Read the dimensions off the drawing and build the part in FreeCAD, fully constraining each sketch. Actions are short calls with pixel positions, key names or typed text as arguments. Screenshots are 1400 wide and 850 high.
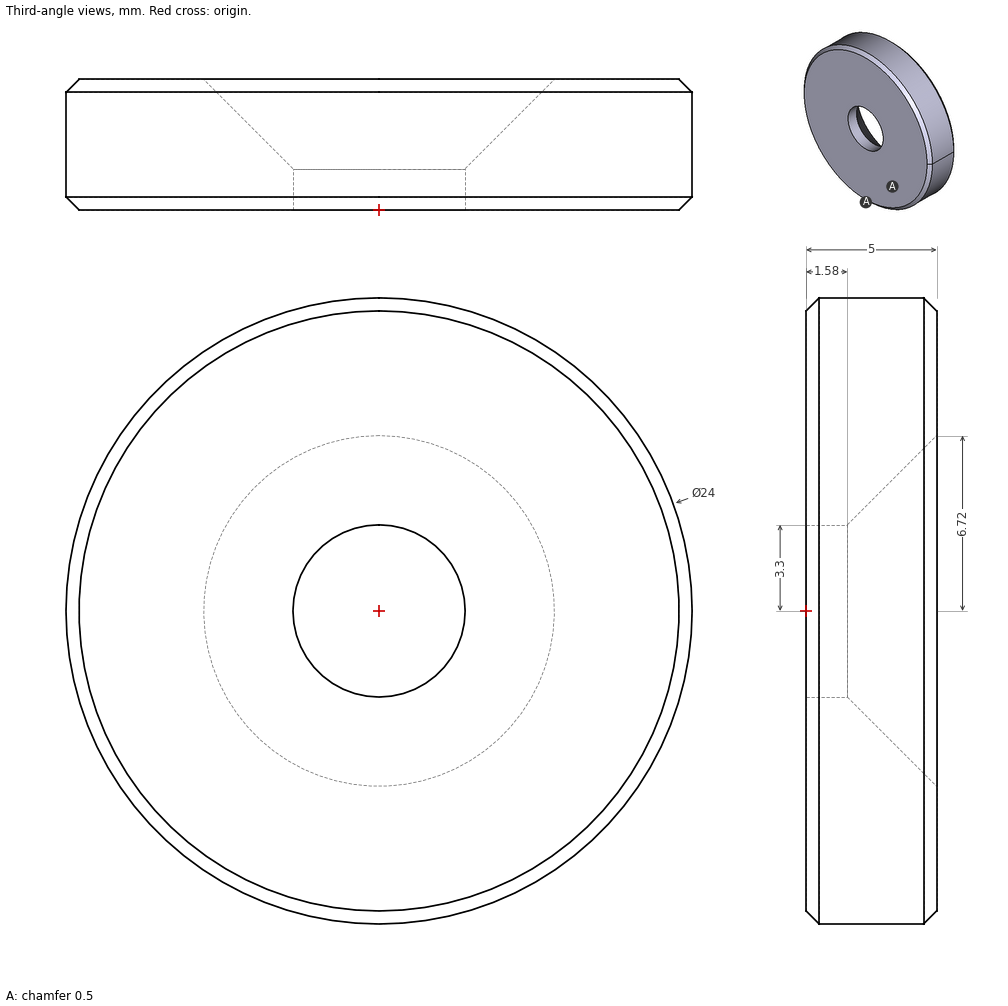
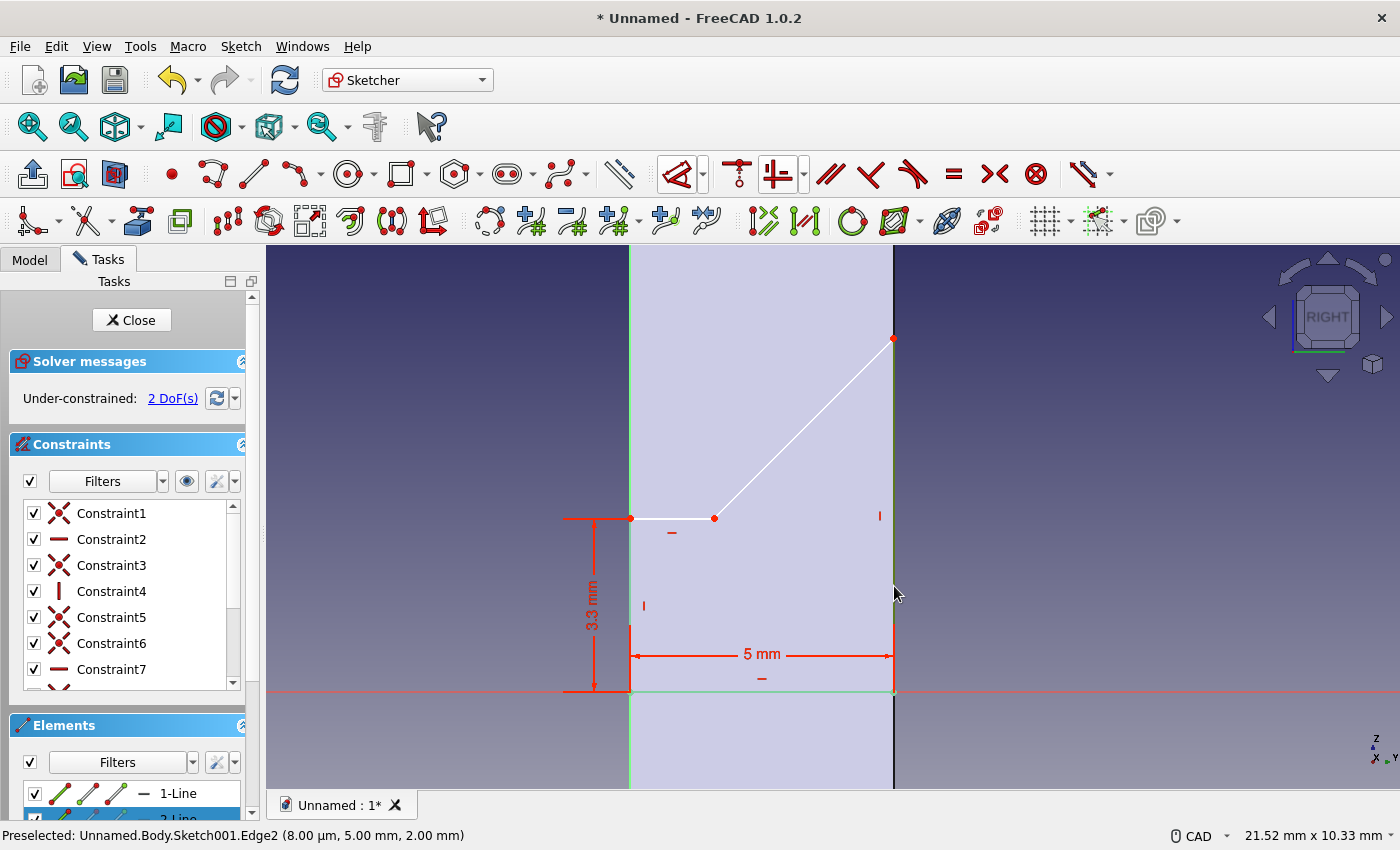
key(i)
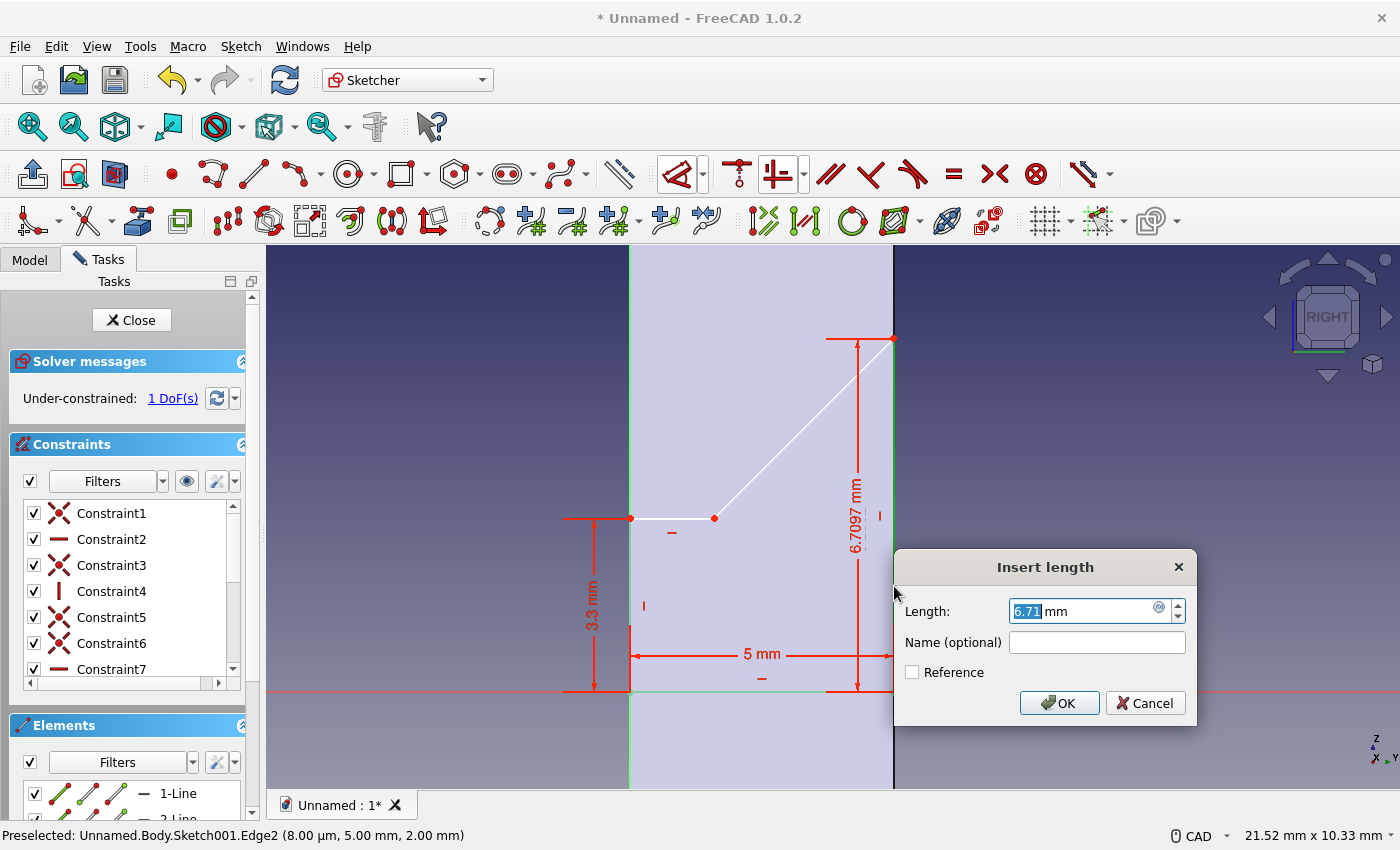
text(6.72)
key(Return)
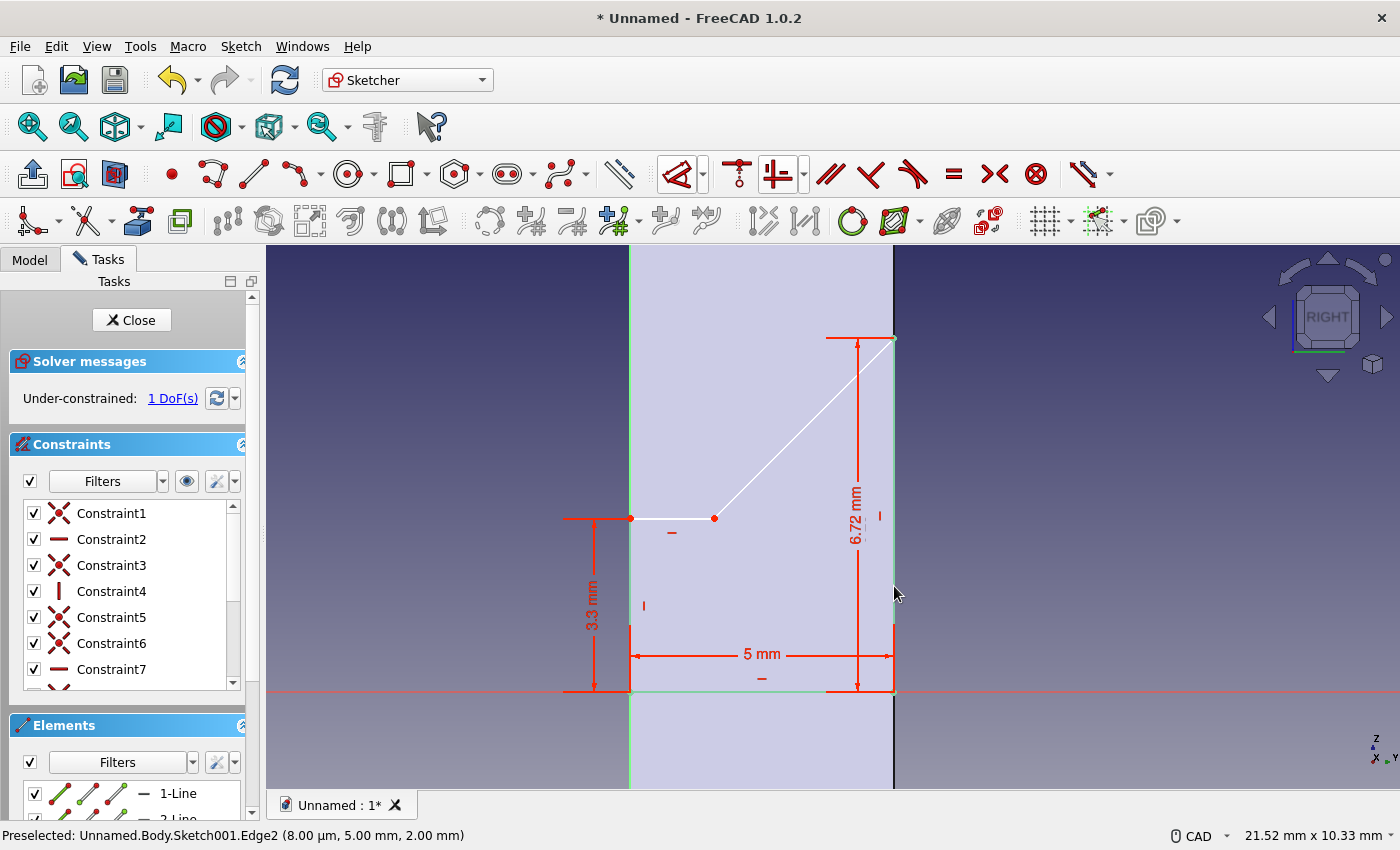
click(689, 519)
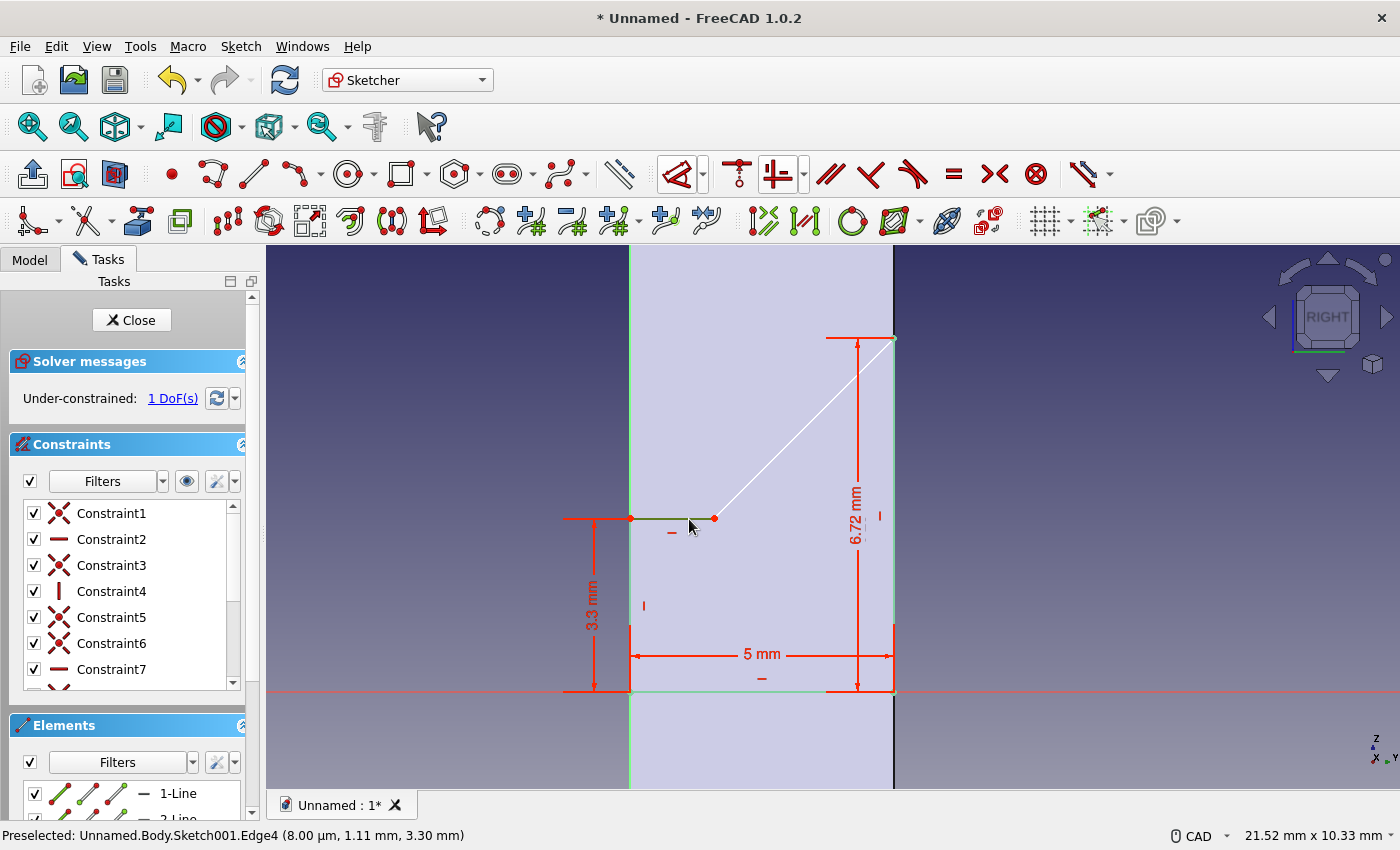
click(702, 174)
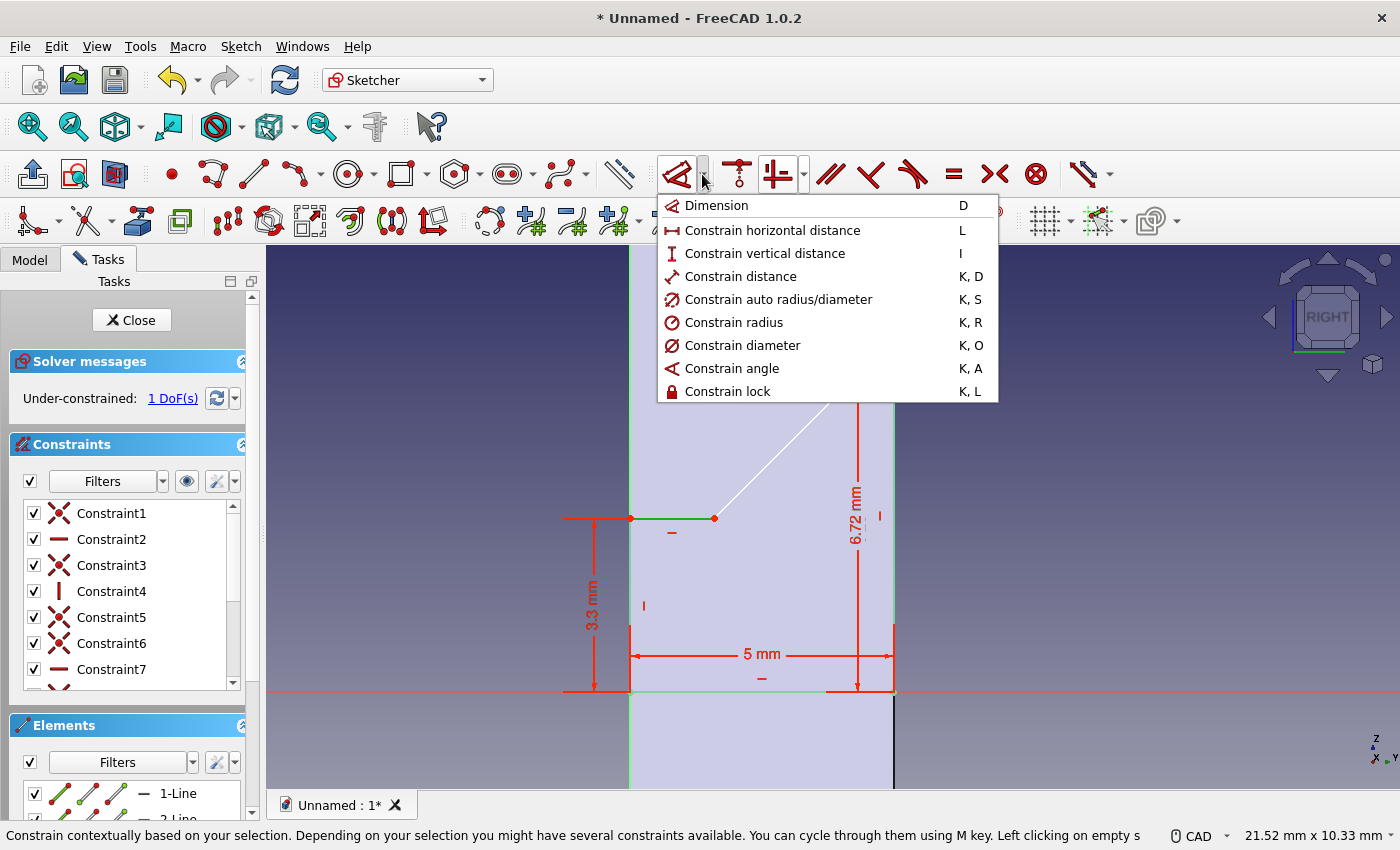
click(828, 230)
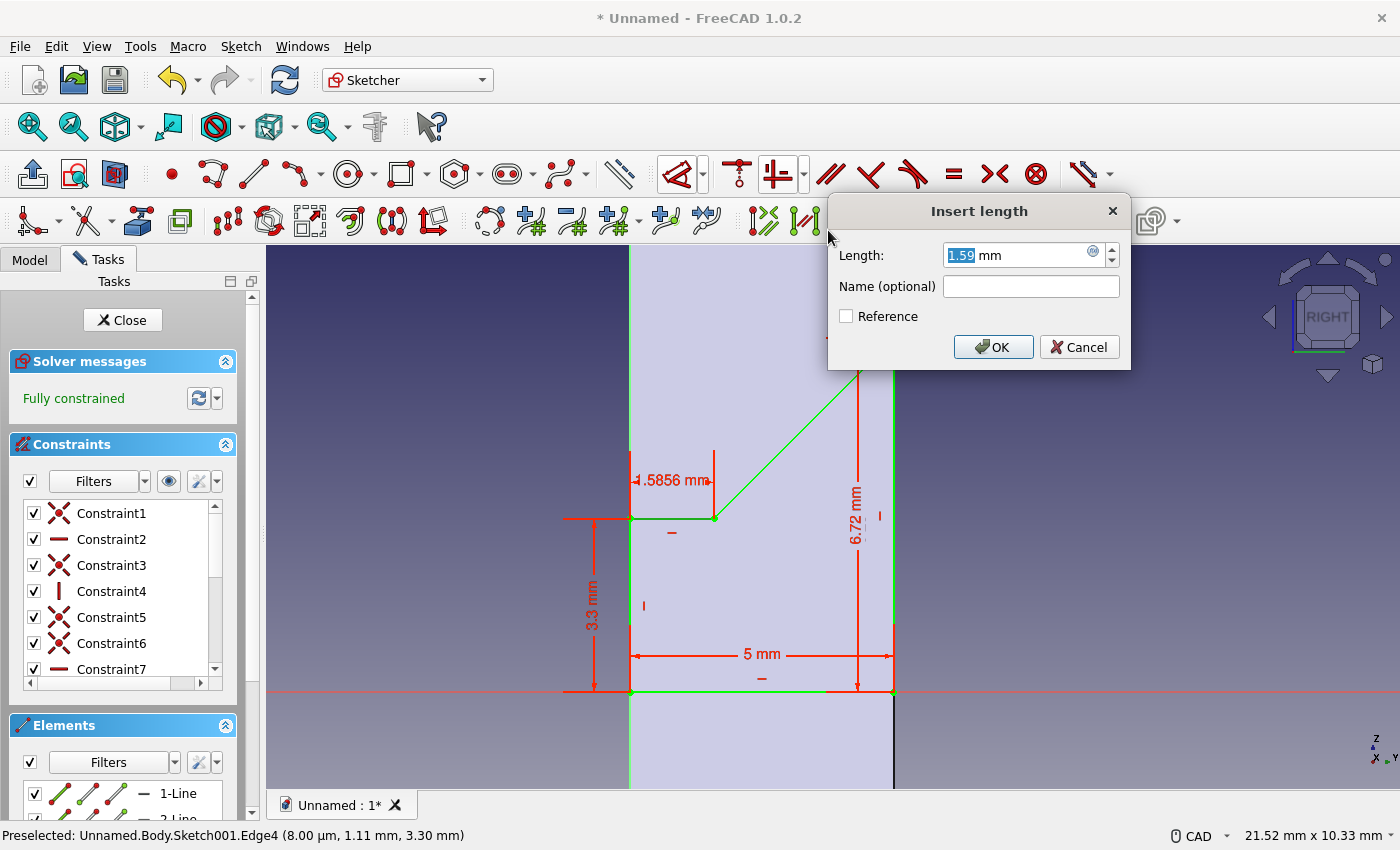
text(1.58)
key(Return)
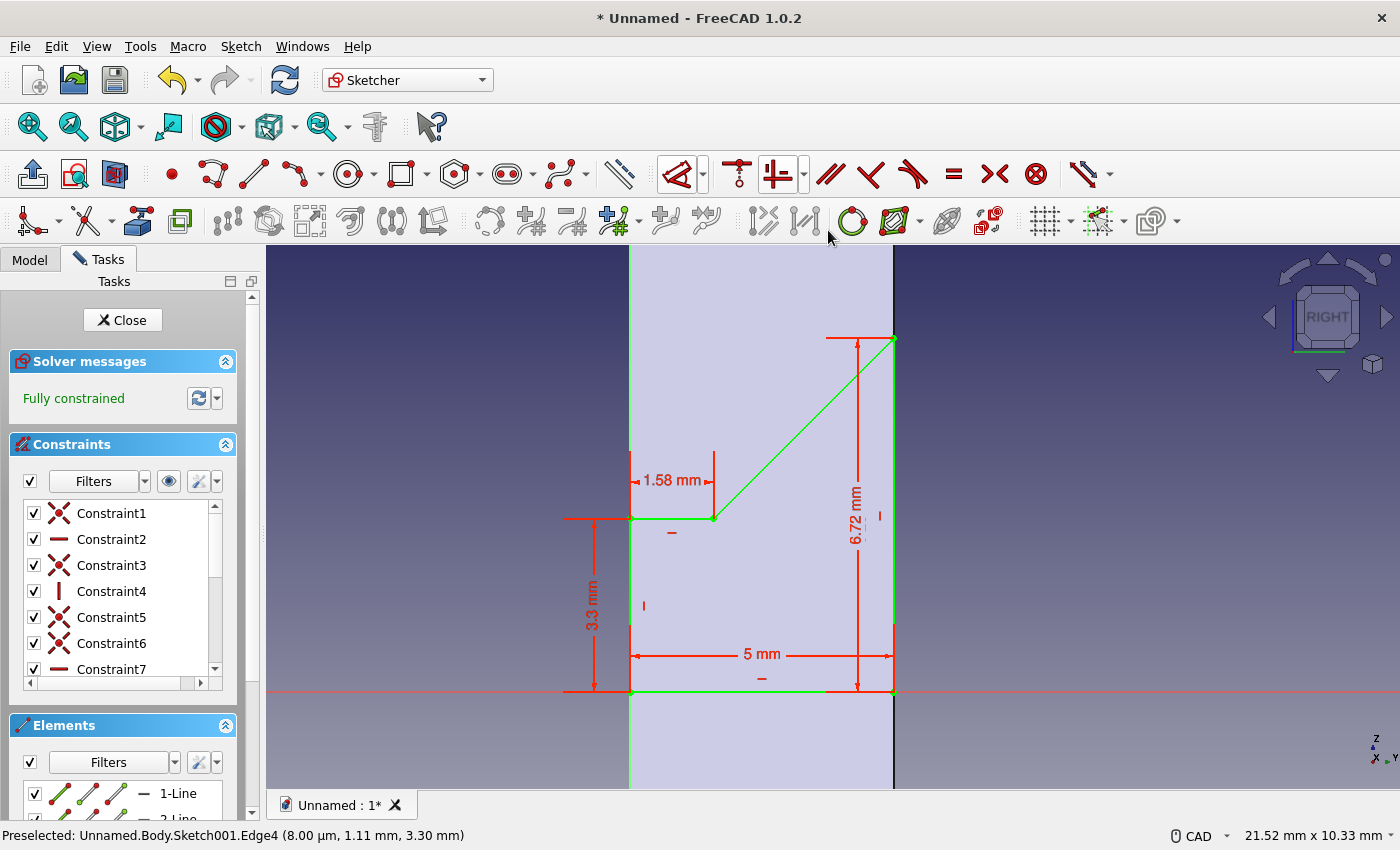
click(123, 320)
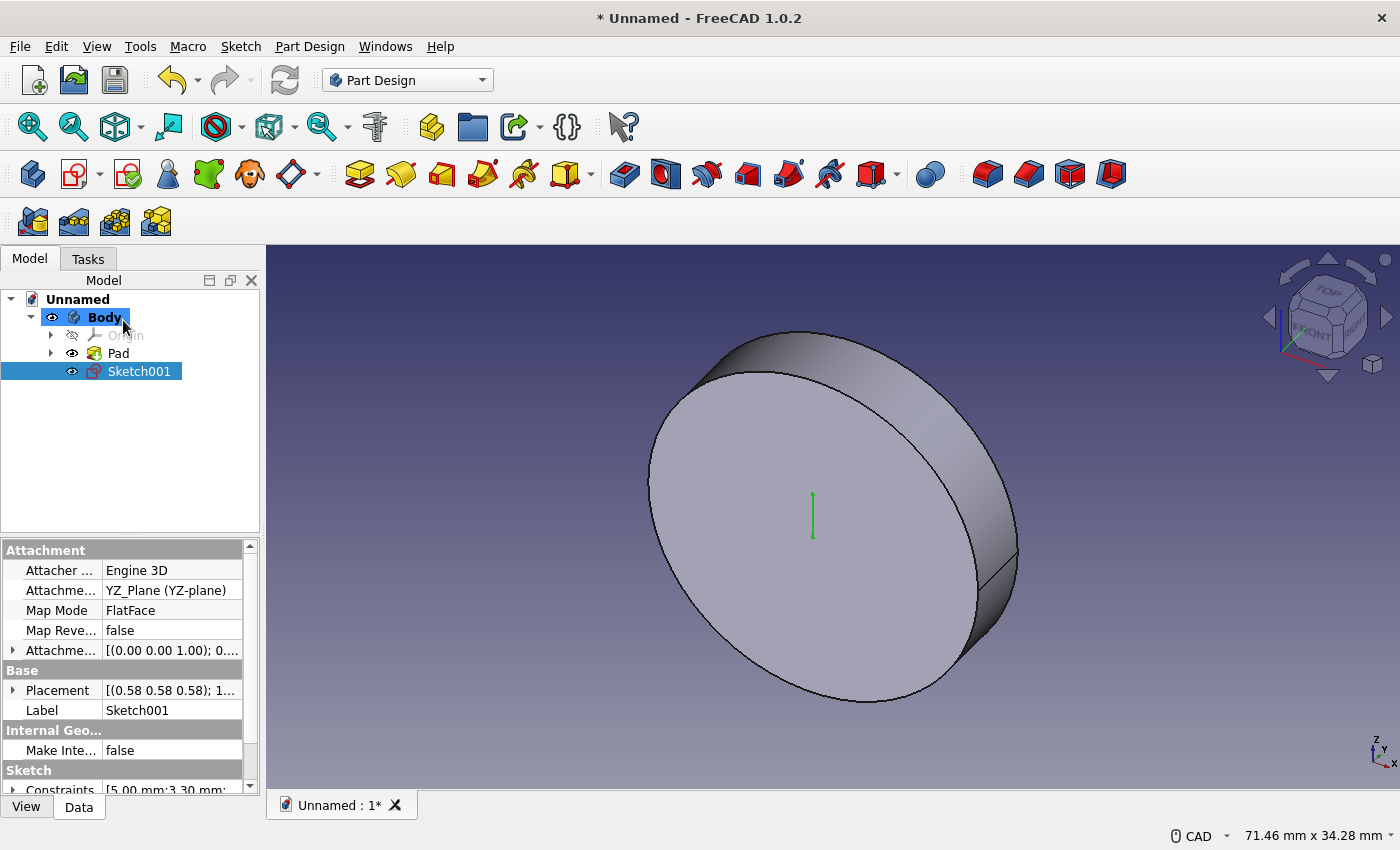
click(707, 174)